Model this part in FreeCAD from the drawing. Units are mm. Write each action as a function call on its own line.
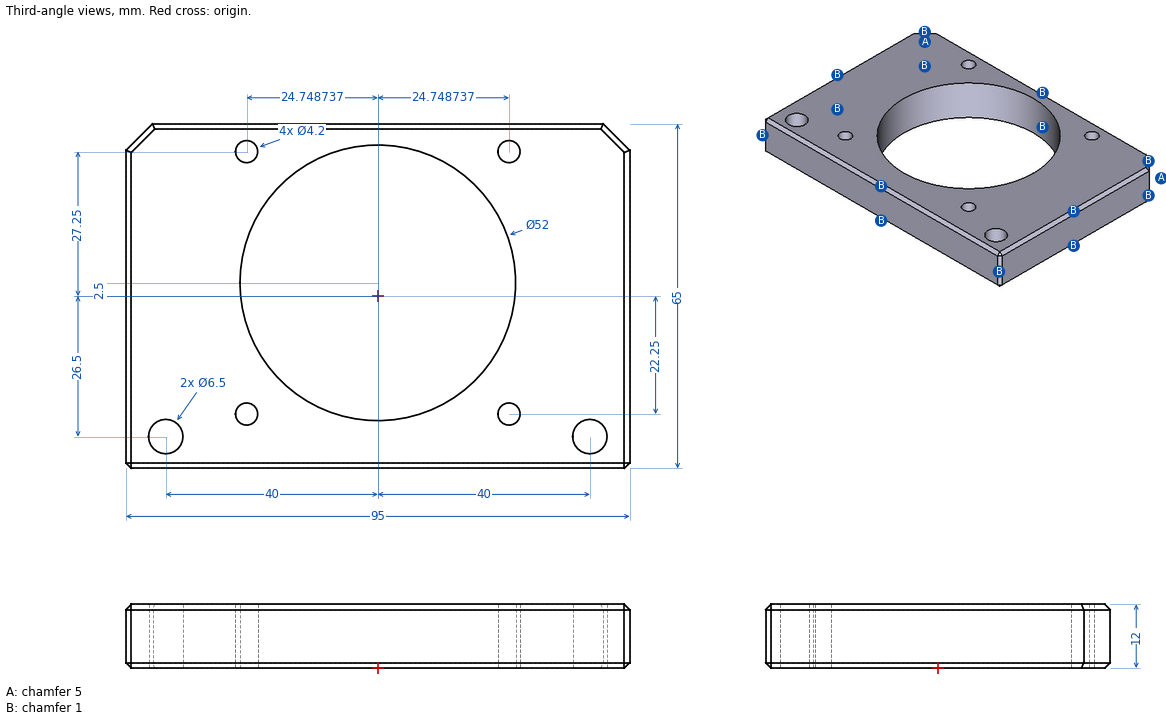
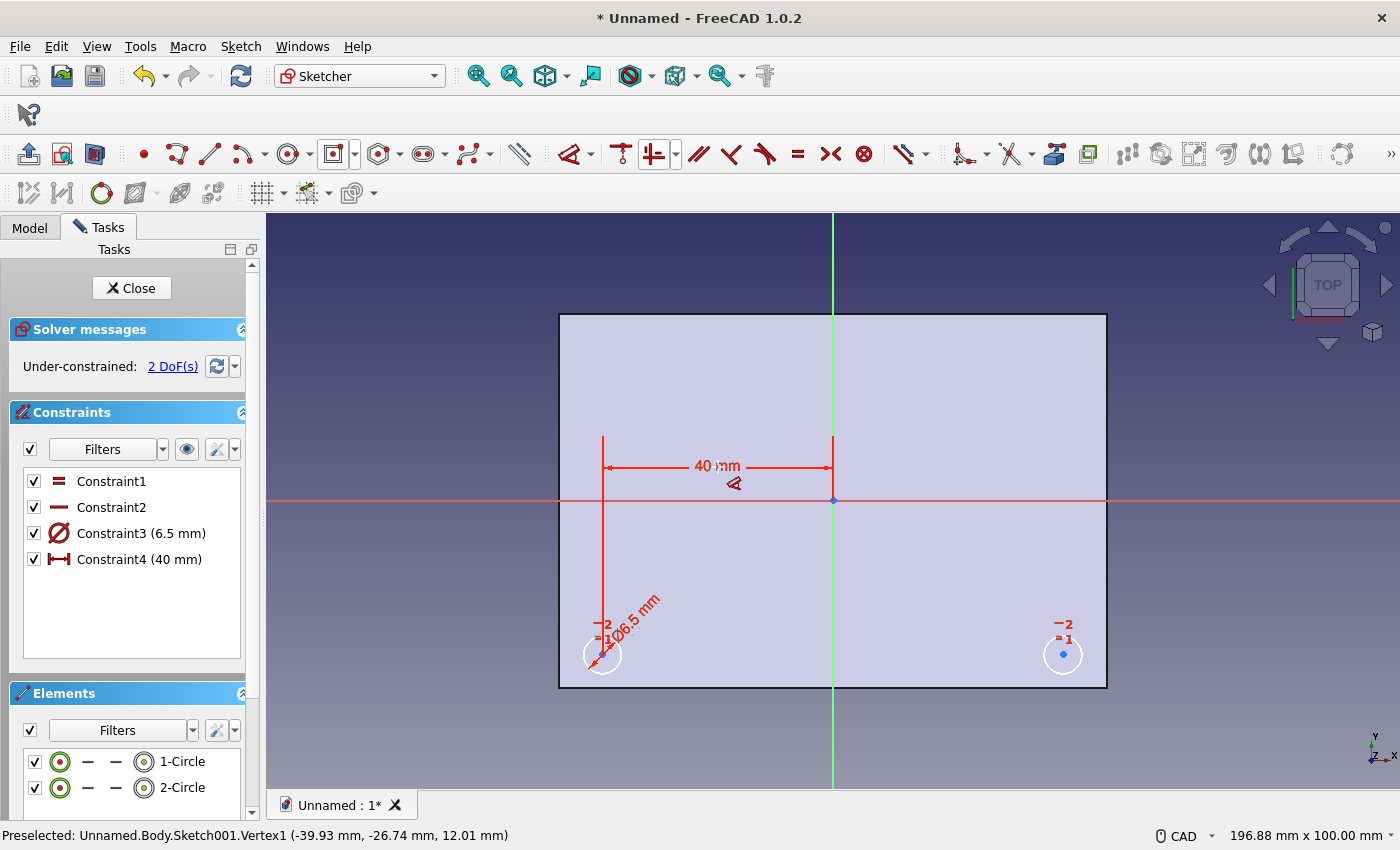
click(1063, 655)
click(948, 467)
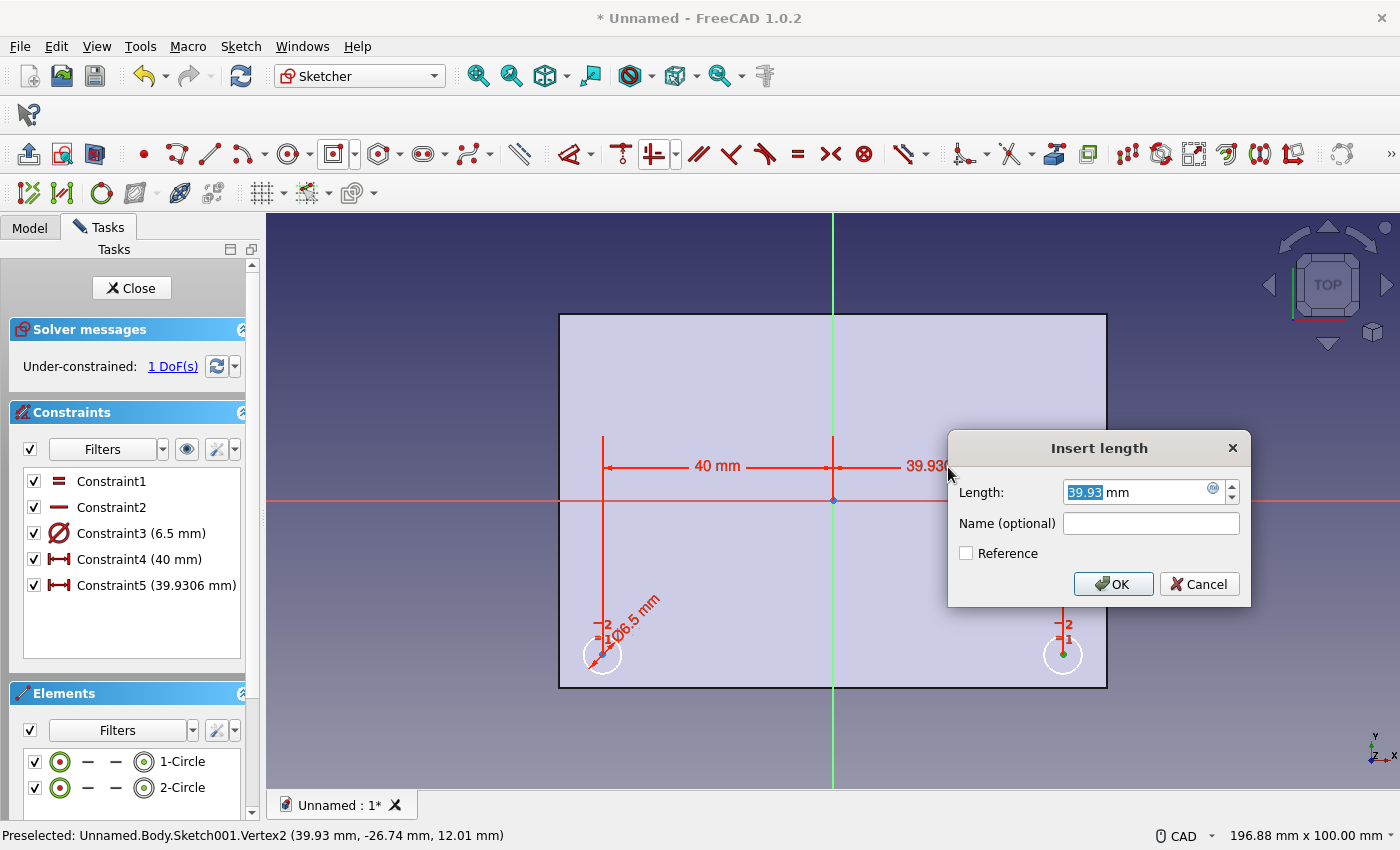
text(40)
key(Return)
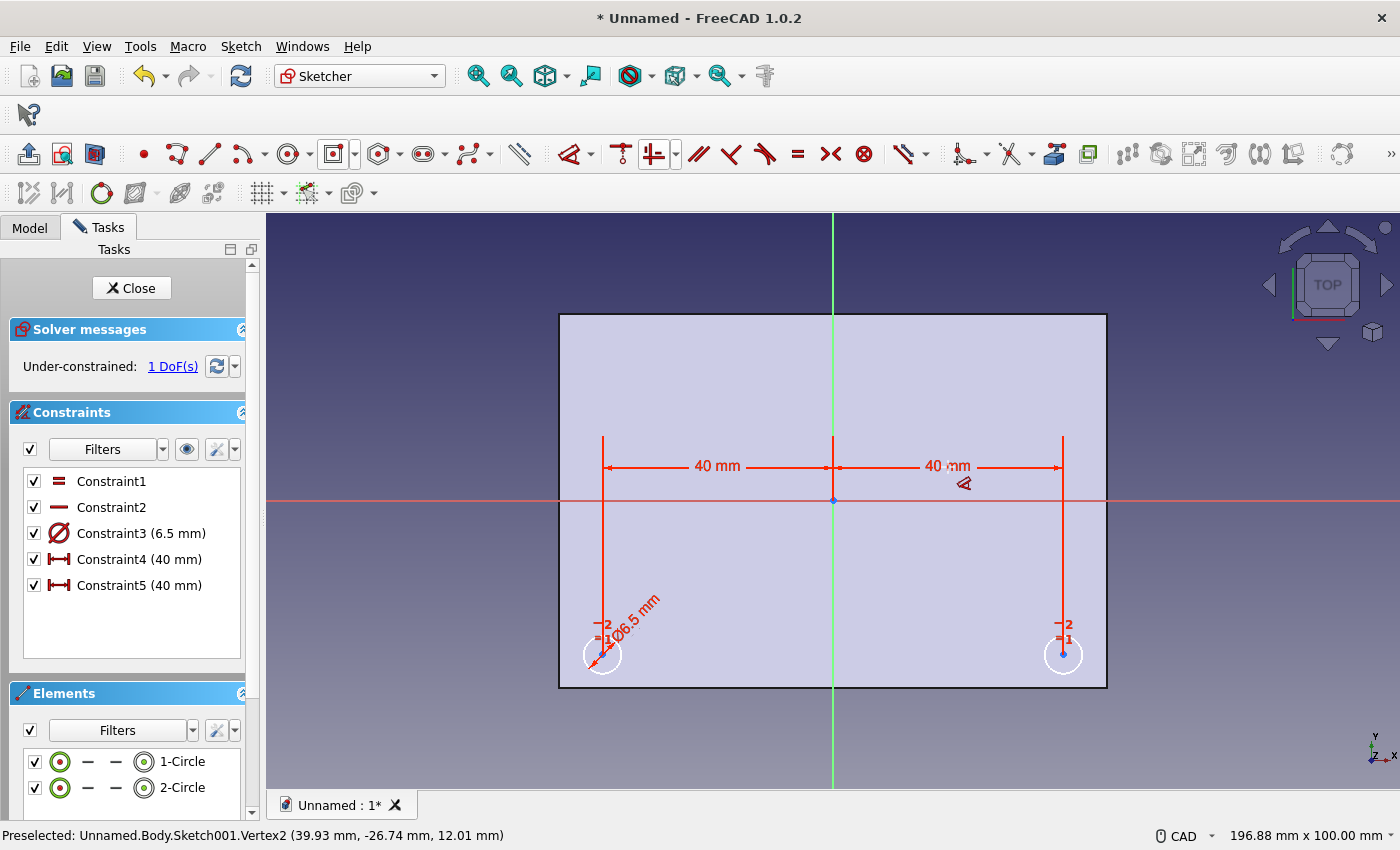
click(603, 655)
click(569, 578)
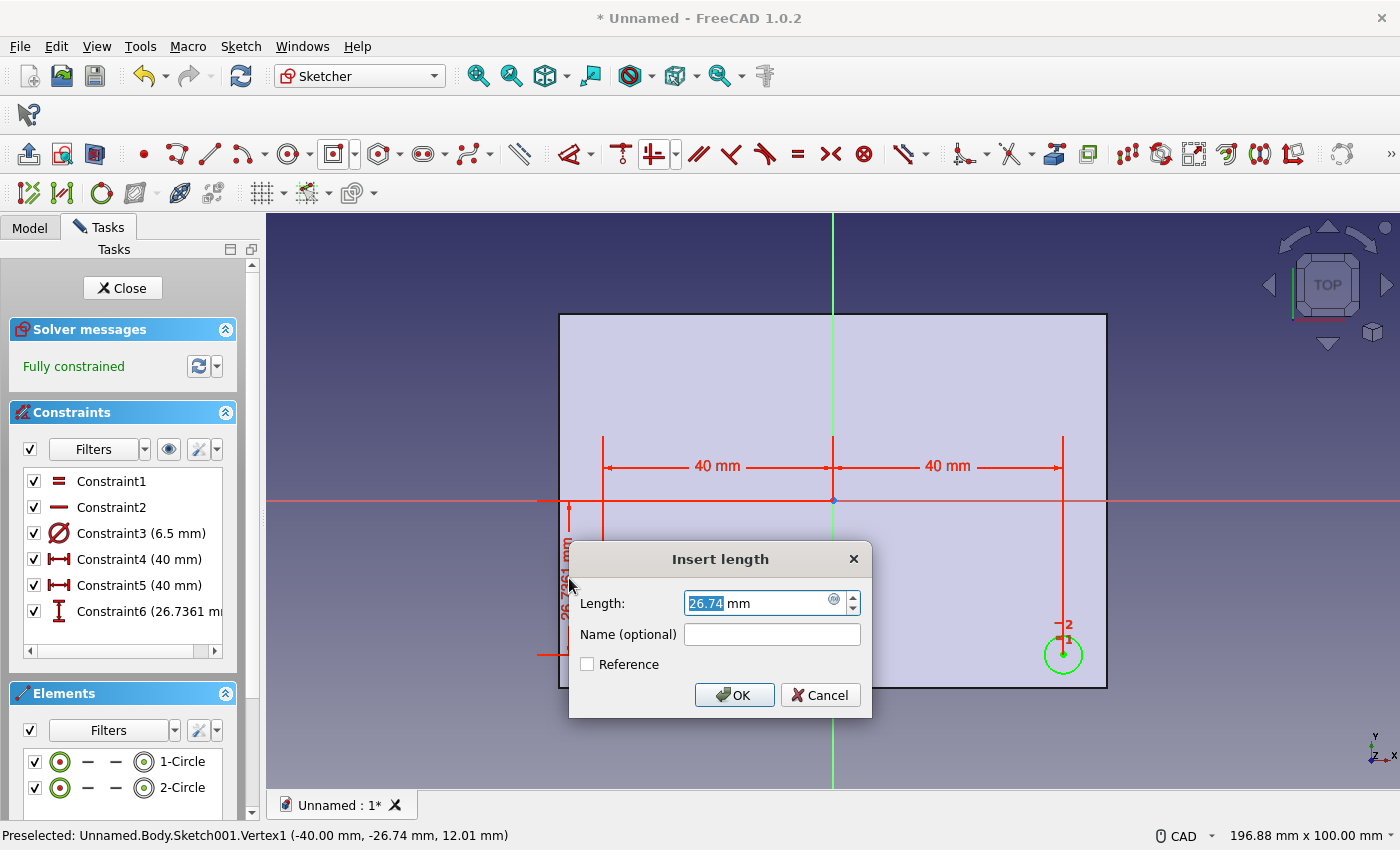
text(26.5)
key(Return)
key(Escape)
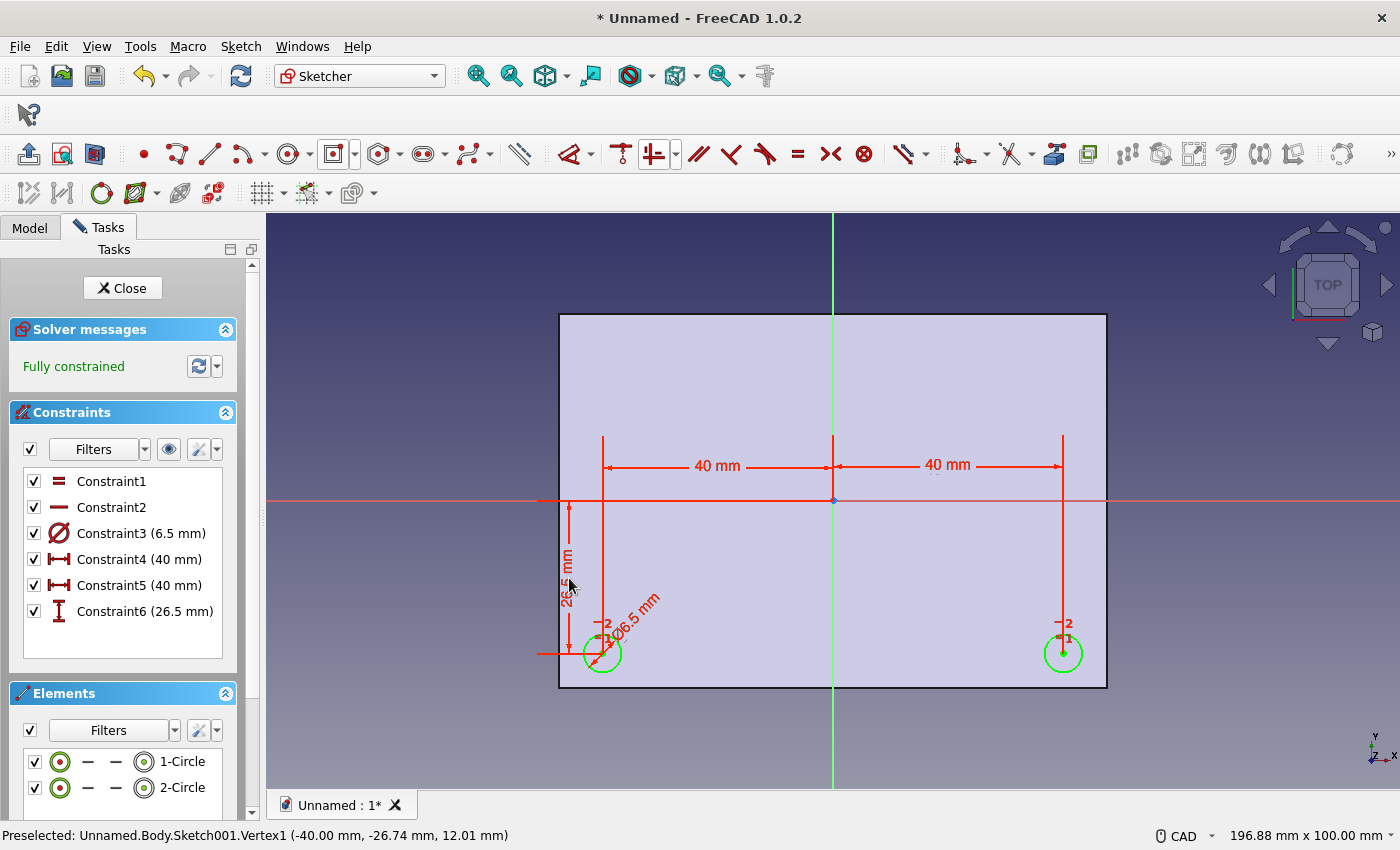
click(123, 288)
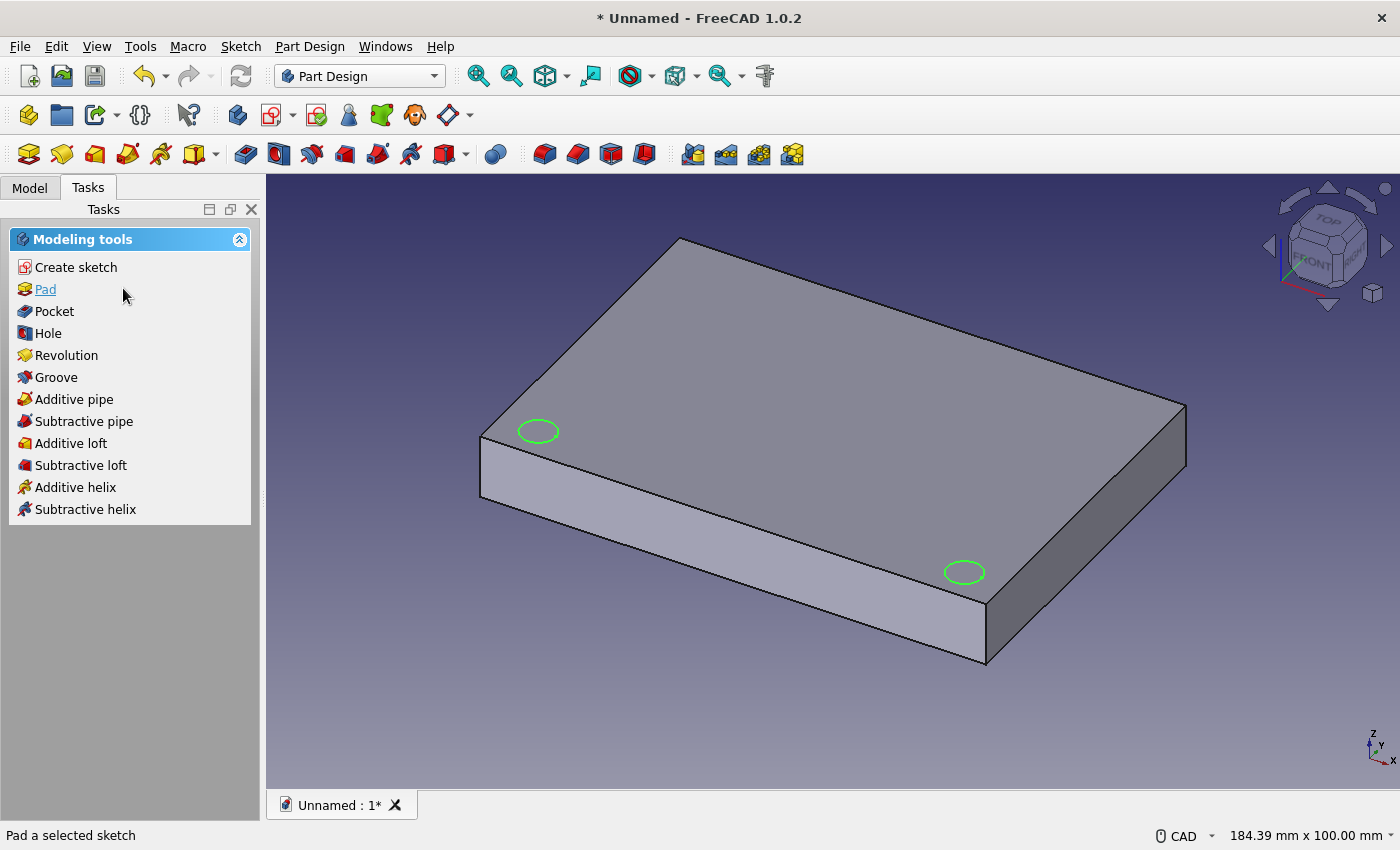
click(246, 154)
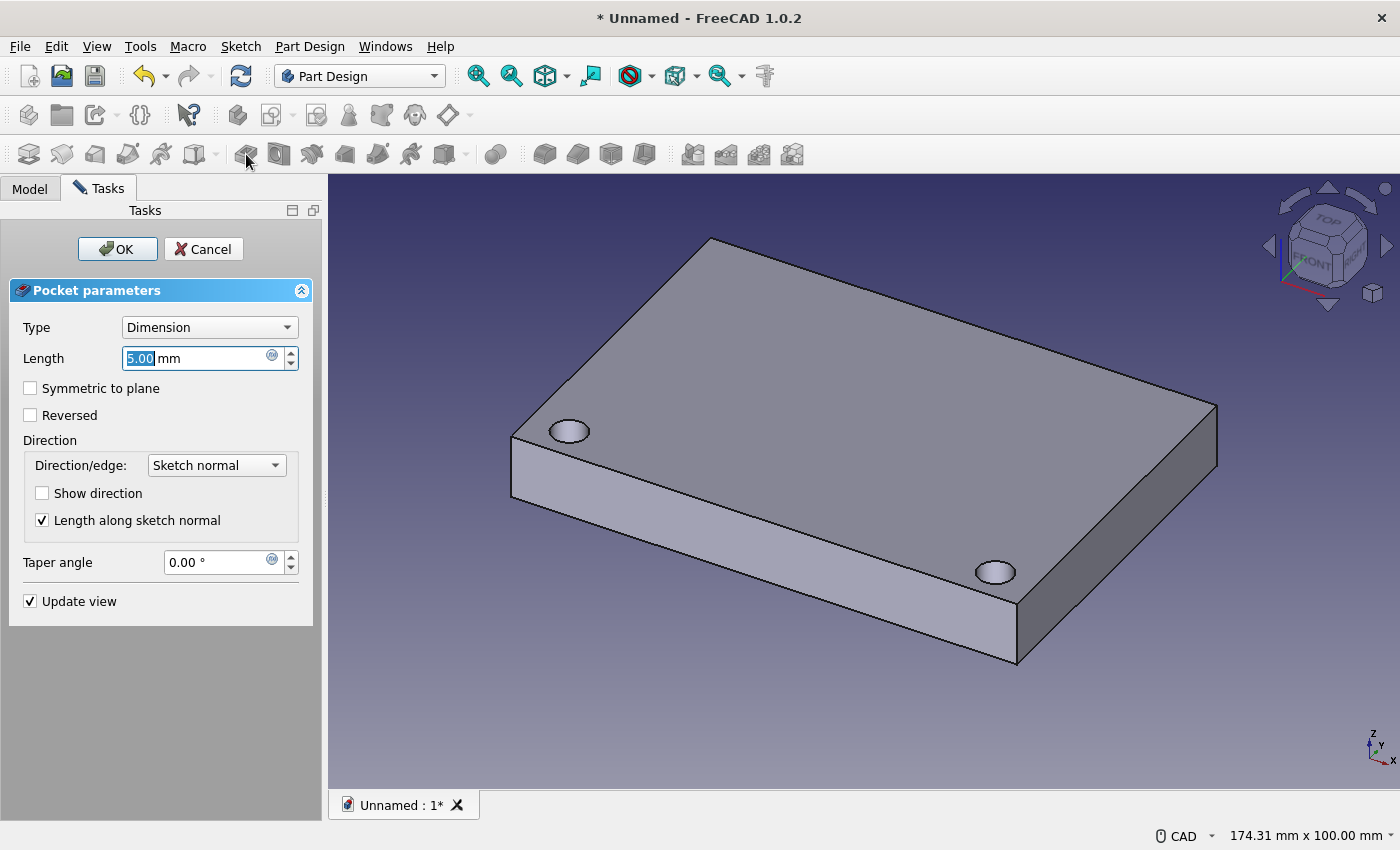
click(210, 328)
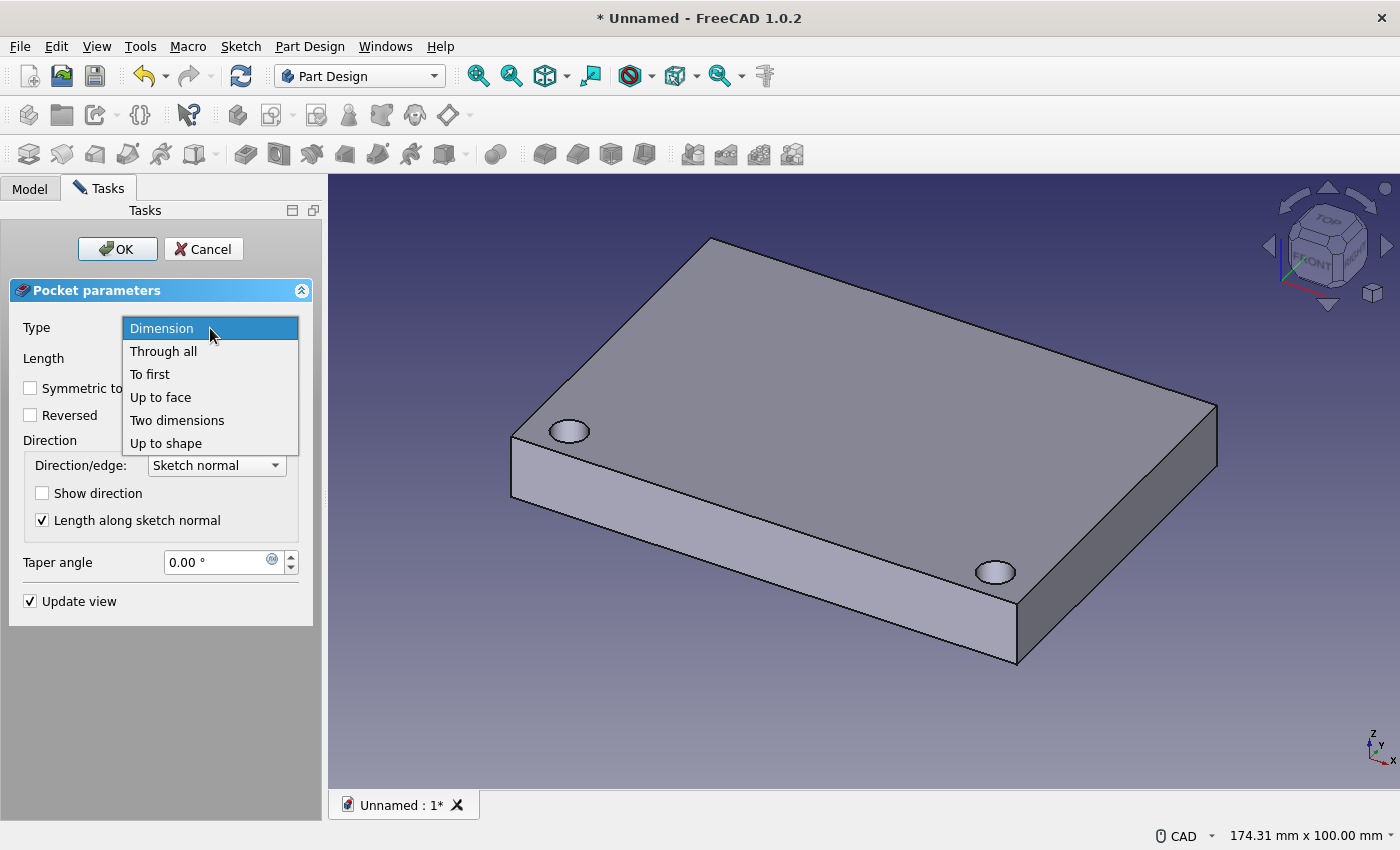
click(208, 352)